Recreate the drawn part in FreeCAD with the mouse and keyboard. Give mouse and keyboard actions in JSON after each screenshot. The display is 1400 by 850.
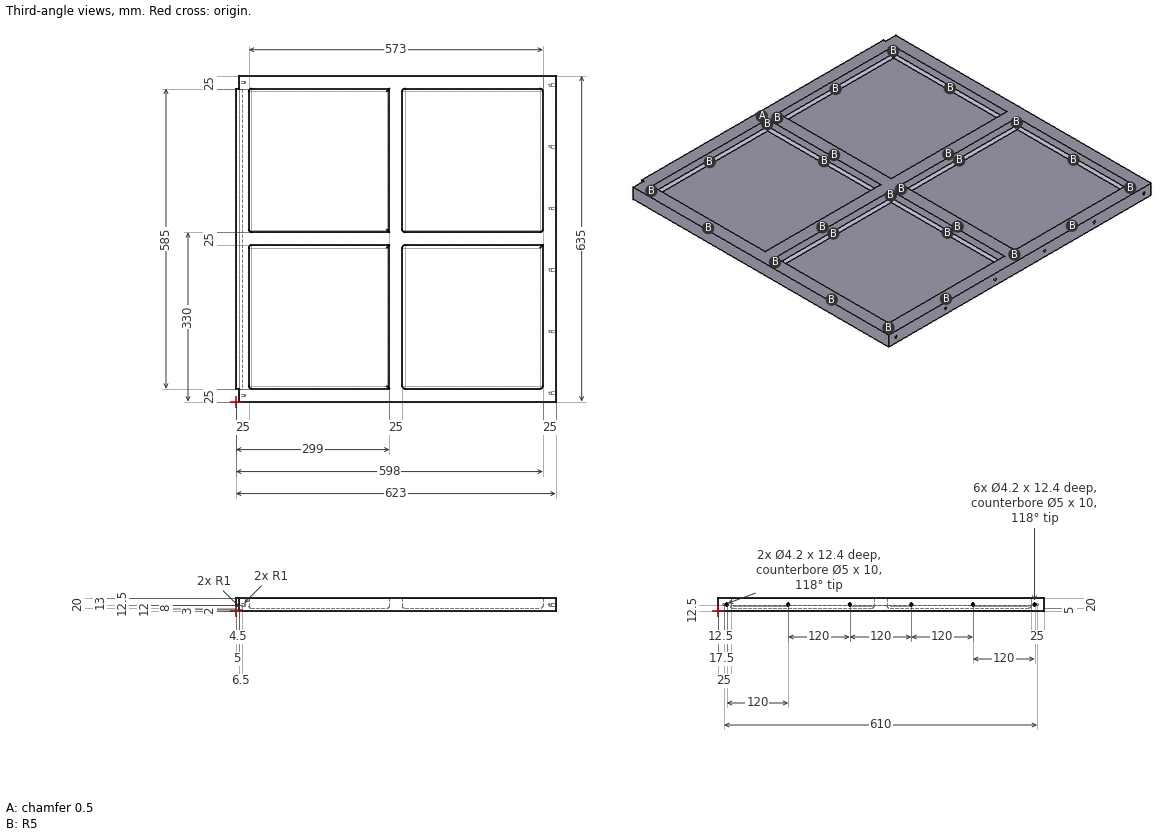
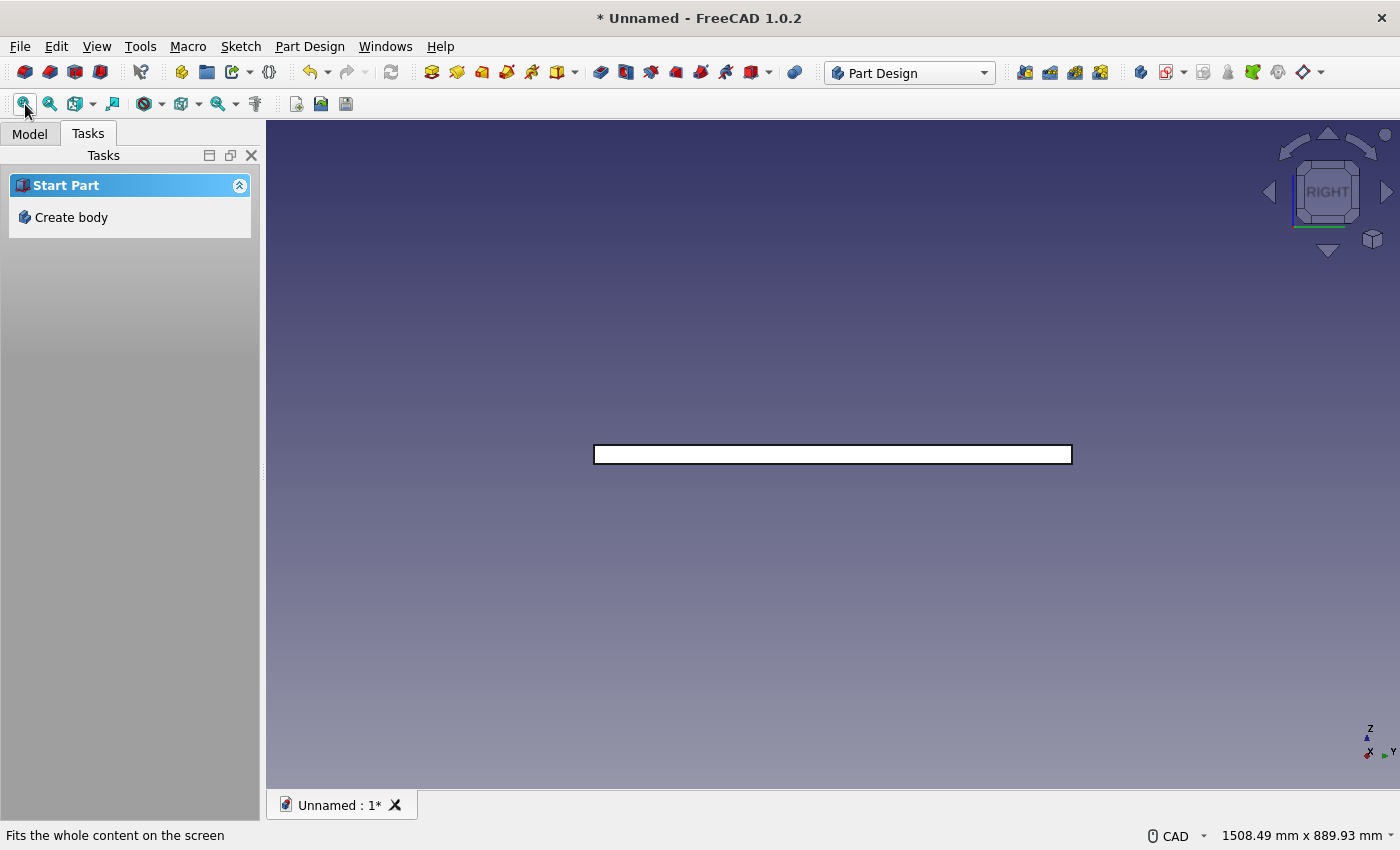
{"action": "key", "text": "5"}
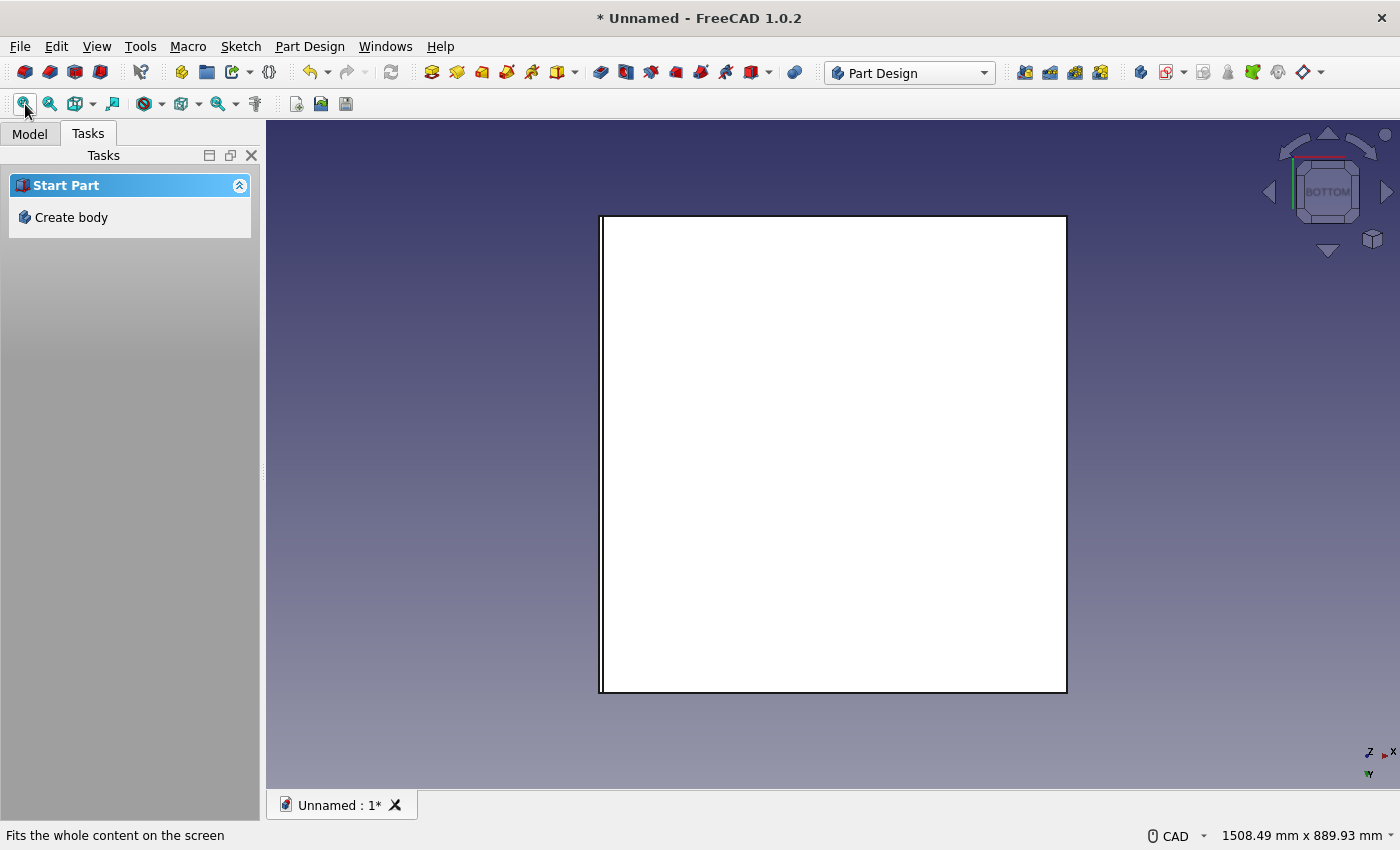
{"action": "key", "text": "4"}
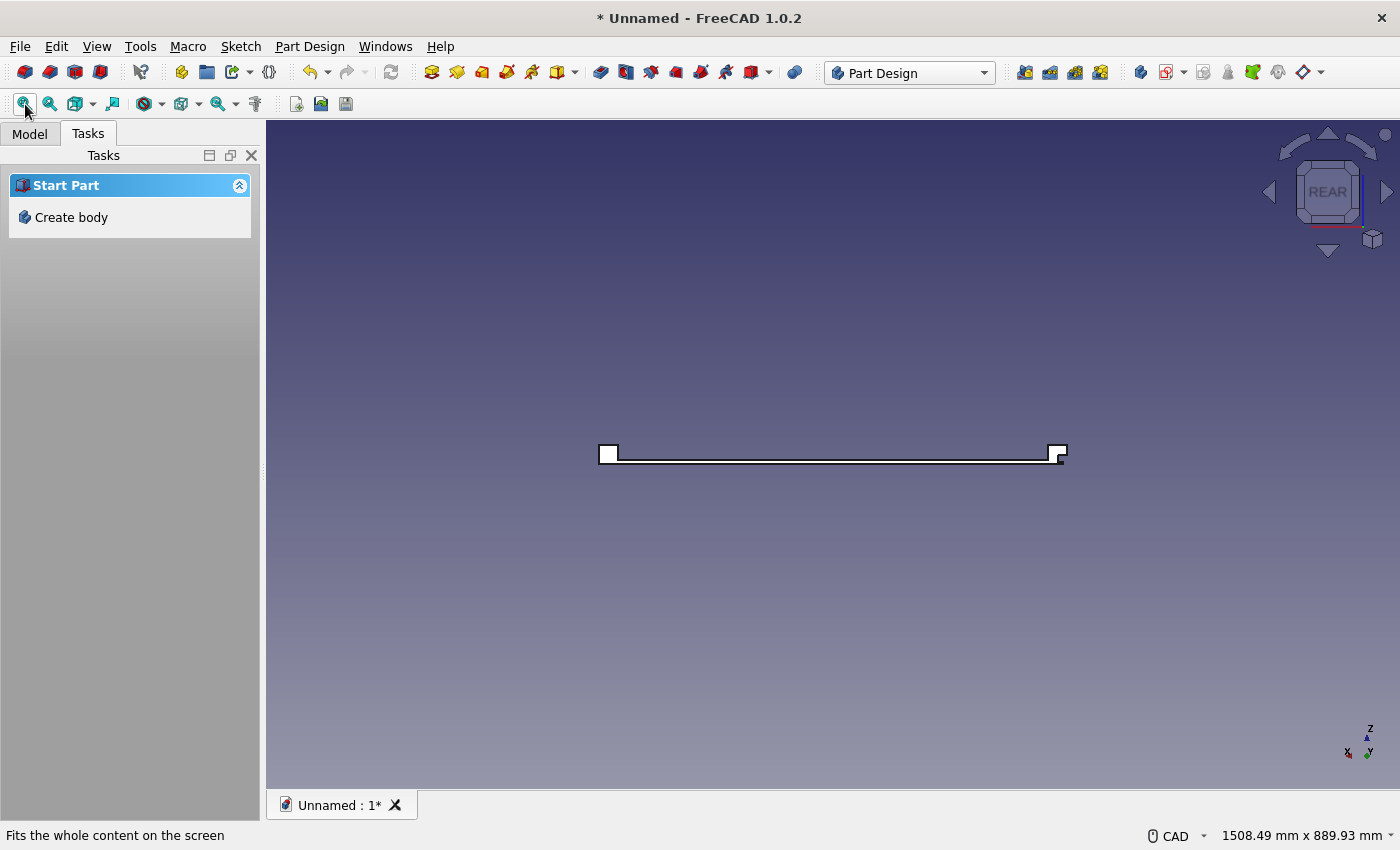
{"action": "left_click", "coordinate": [25, 104]}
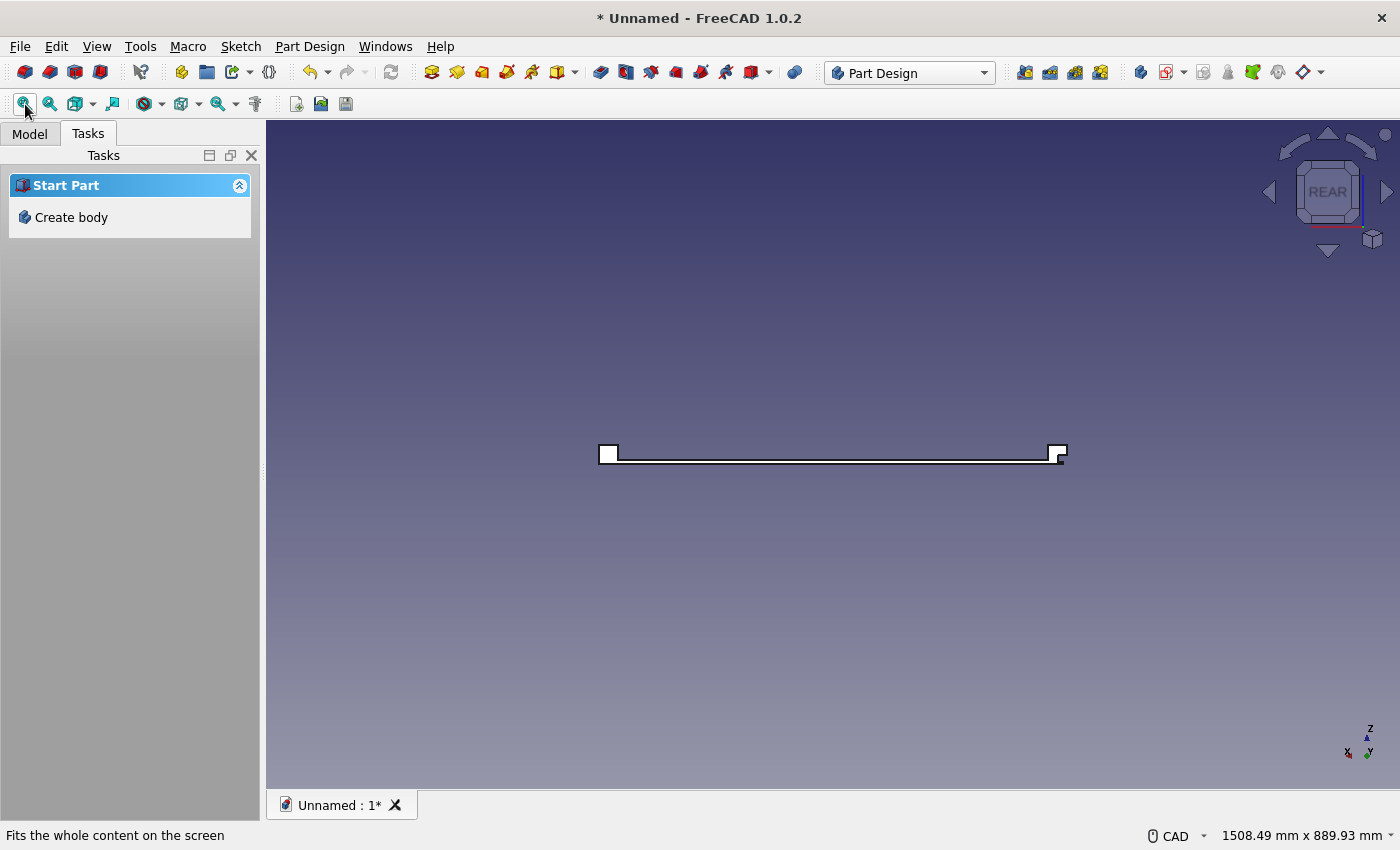
{"action": "key", "text": "6"}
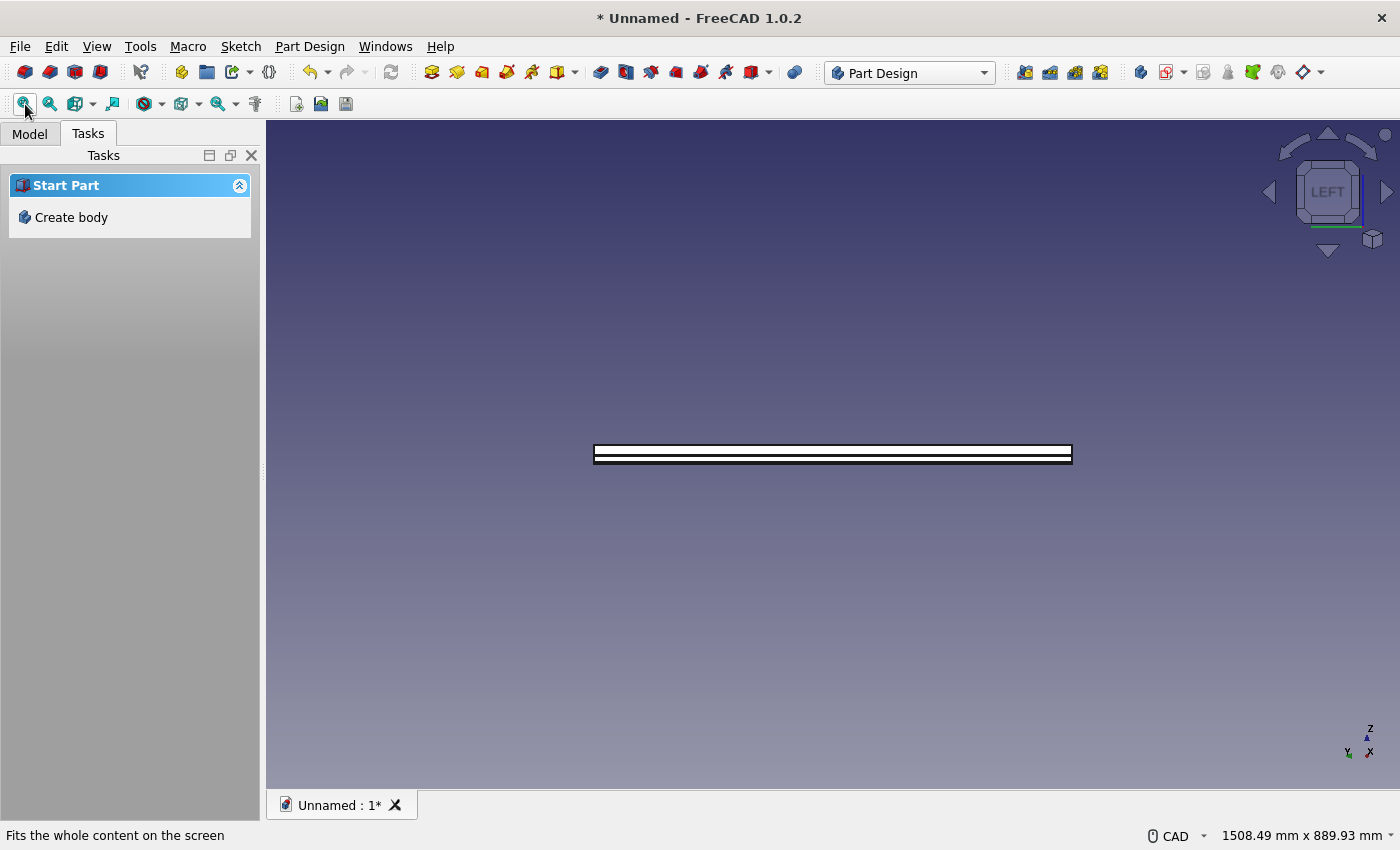
{"action": "key", "text": "v f"}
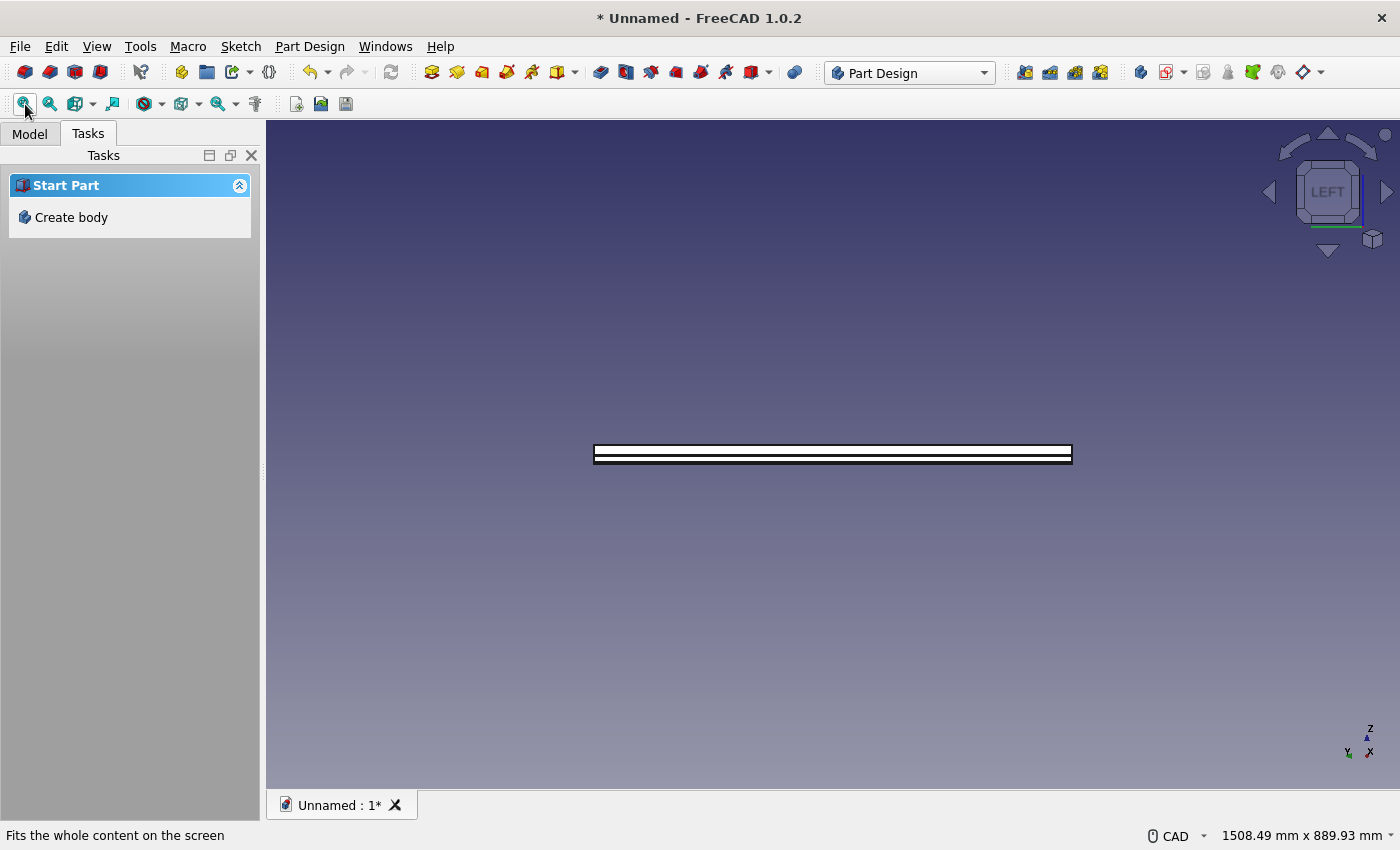
{"action": "left_click", "coordinate": [833, 454]}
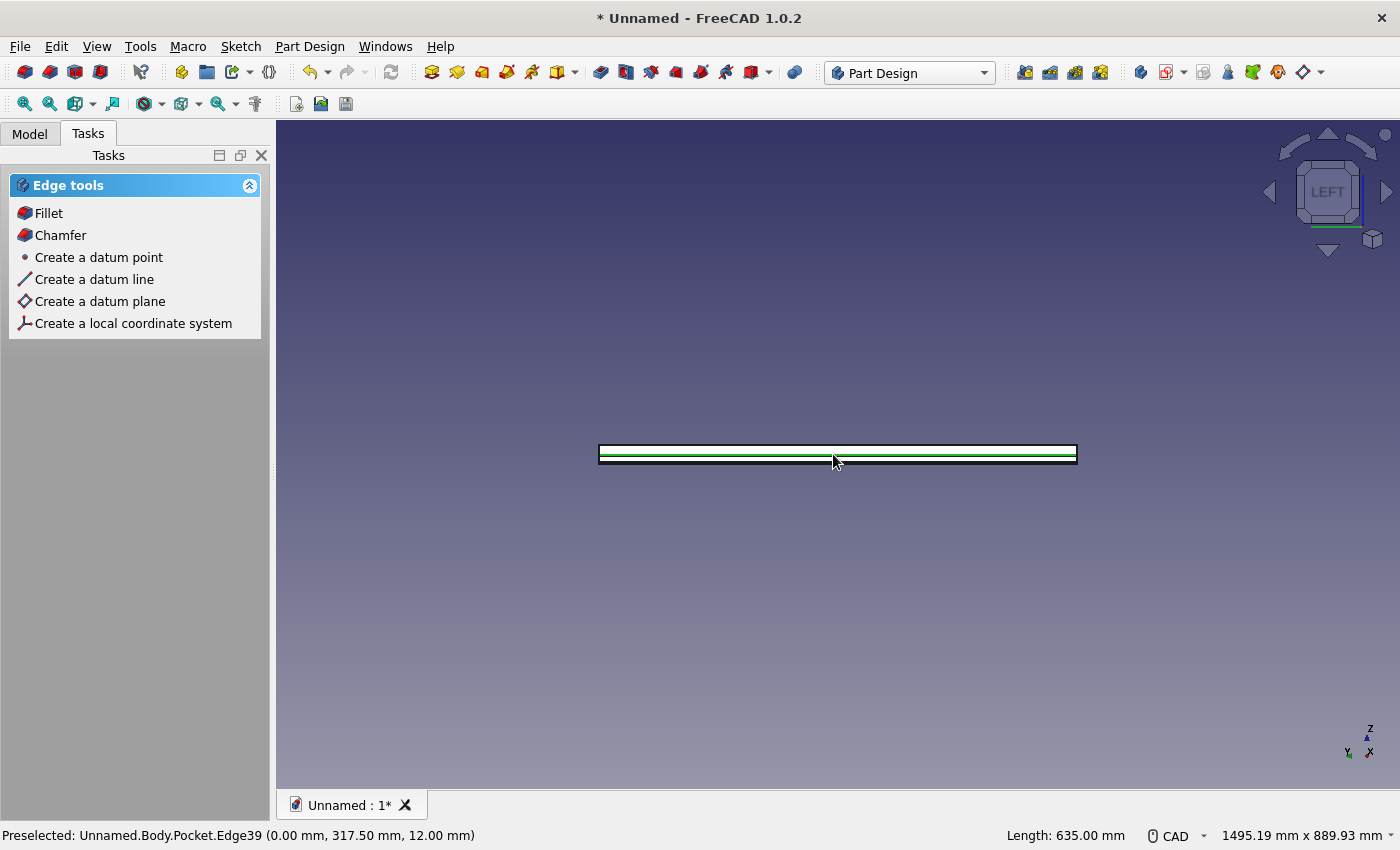
{"action": "left_click", "coordinate": [50, 72]}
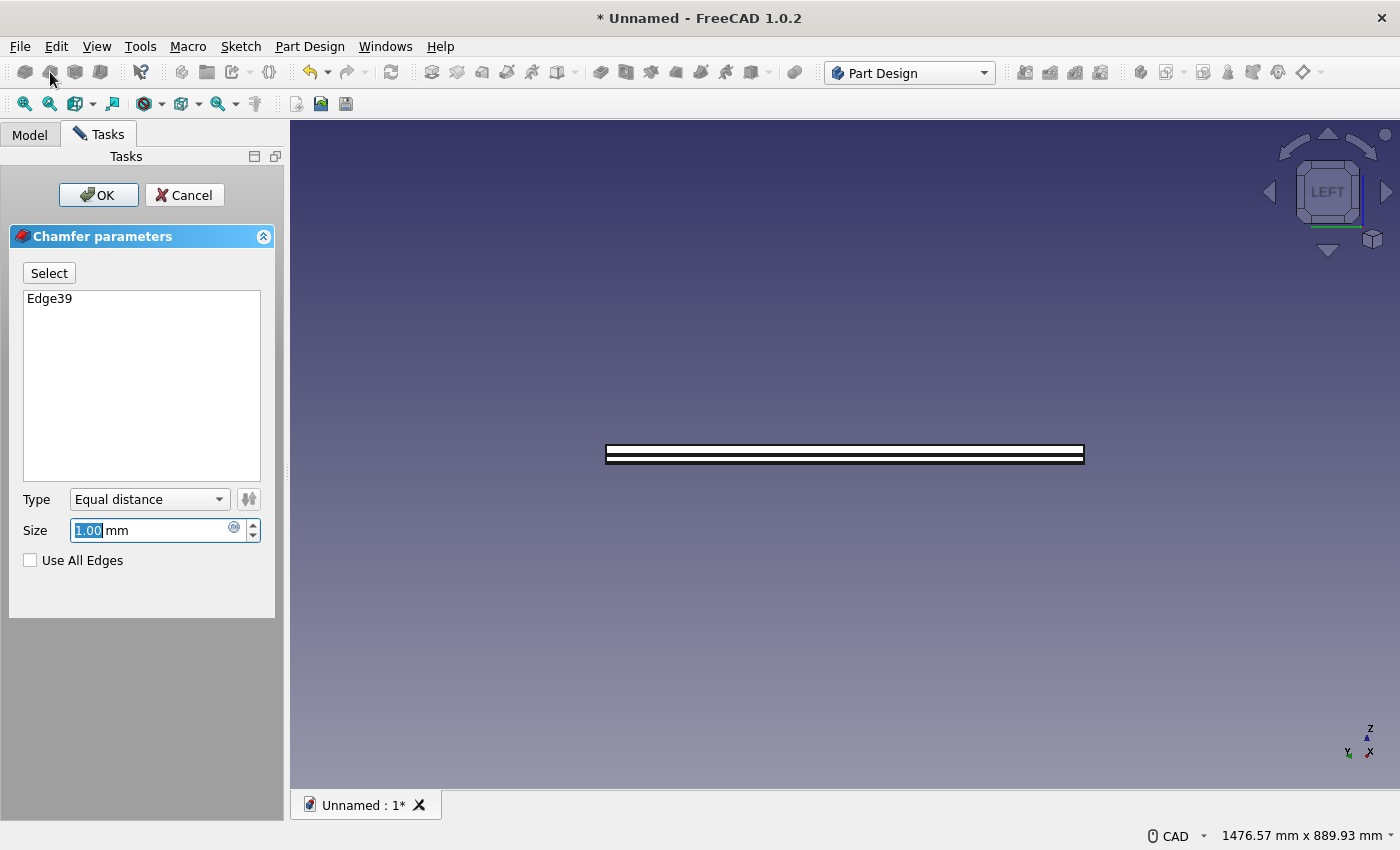
{"action": "type", "text": "0.5"}
{"action": "key", "text": "Tab"}